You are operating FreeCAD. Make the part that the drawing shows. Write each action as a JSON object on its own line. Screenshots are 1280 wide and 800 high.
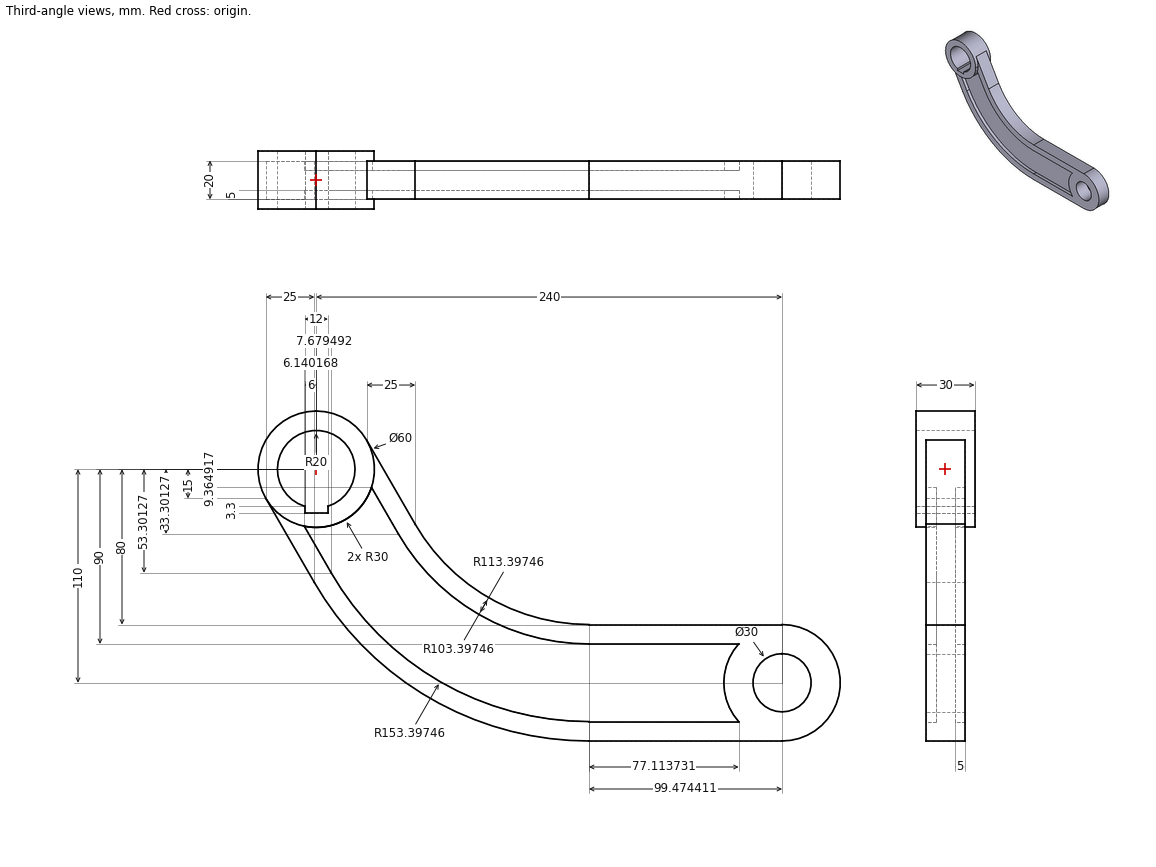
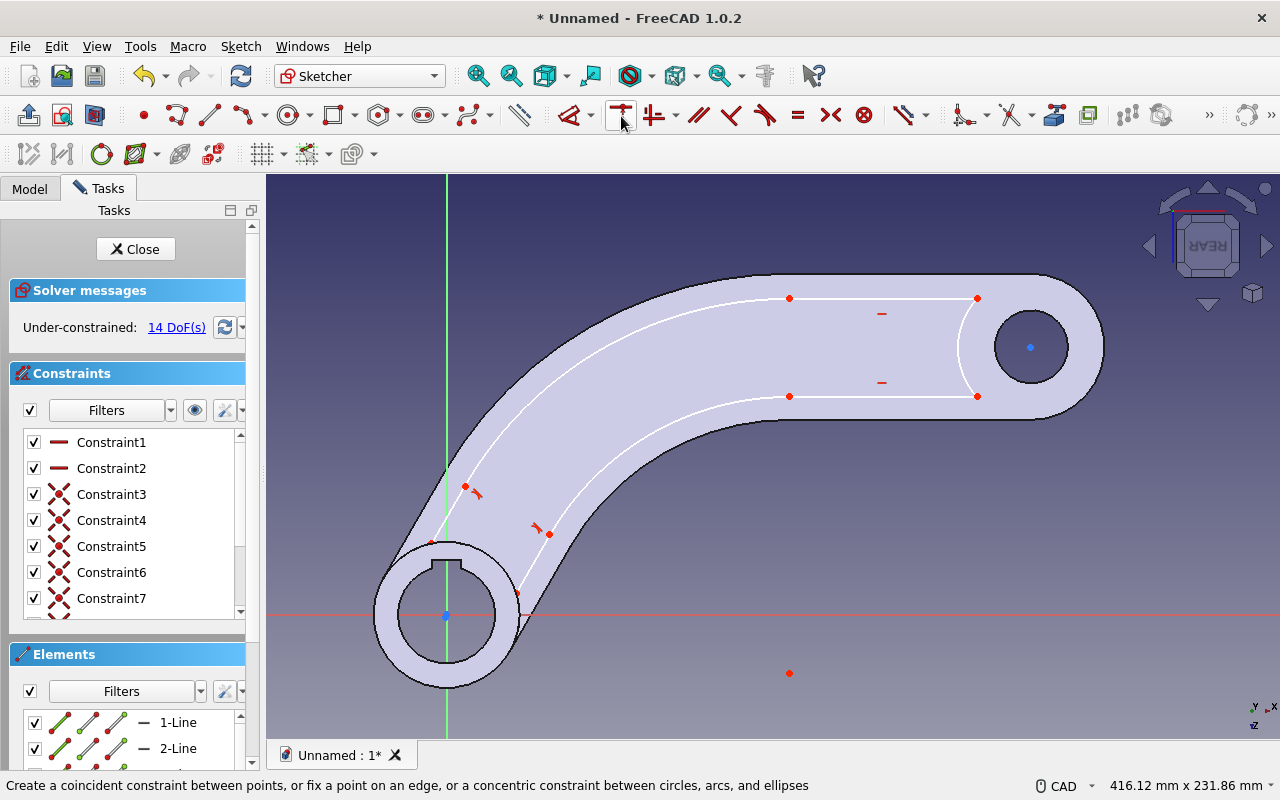
{"action": "left_click_drag", "start_coordinate": [436, 605], "coordinate": [457, 628]}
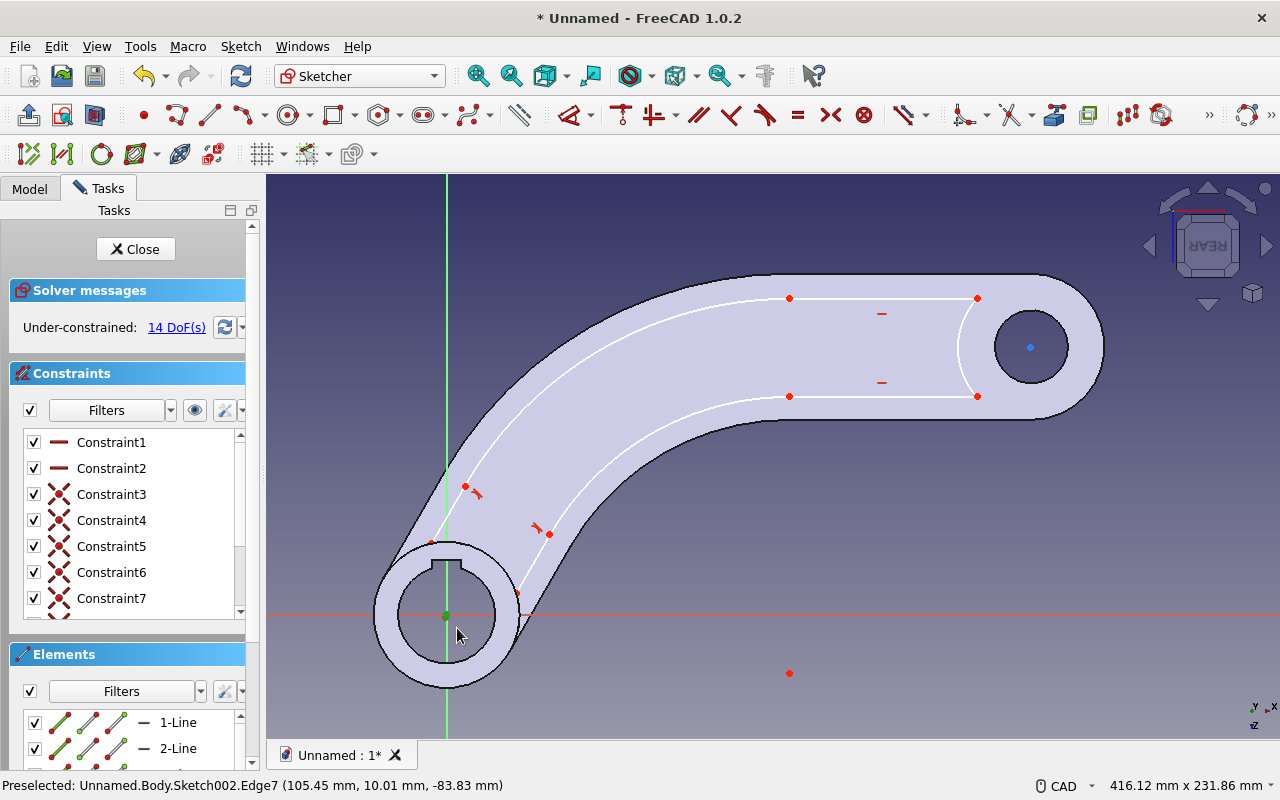
{"action": "left_click", "coordinate": [621, 116]}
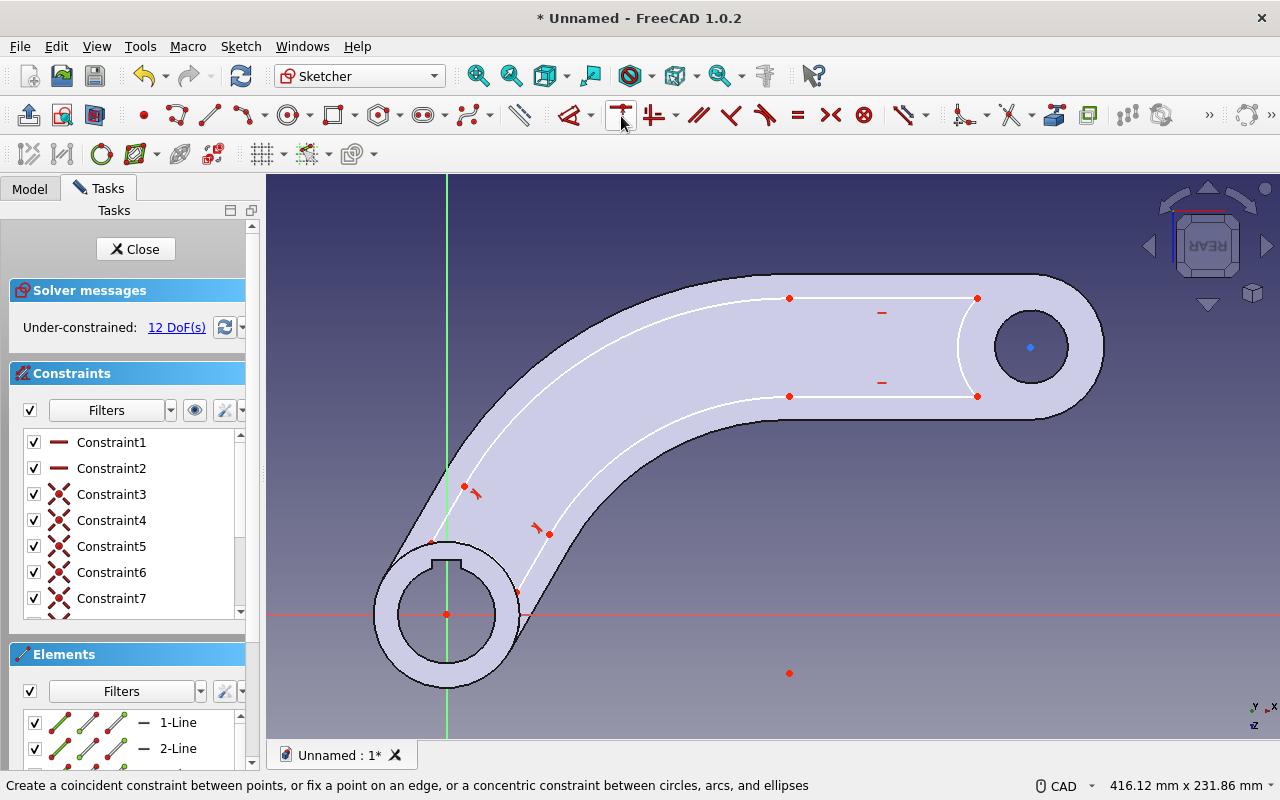
{"action": "left_click", "coordinate": [500, 565]}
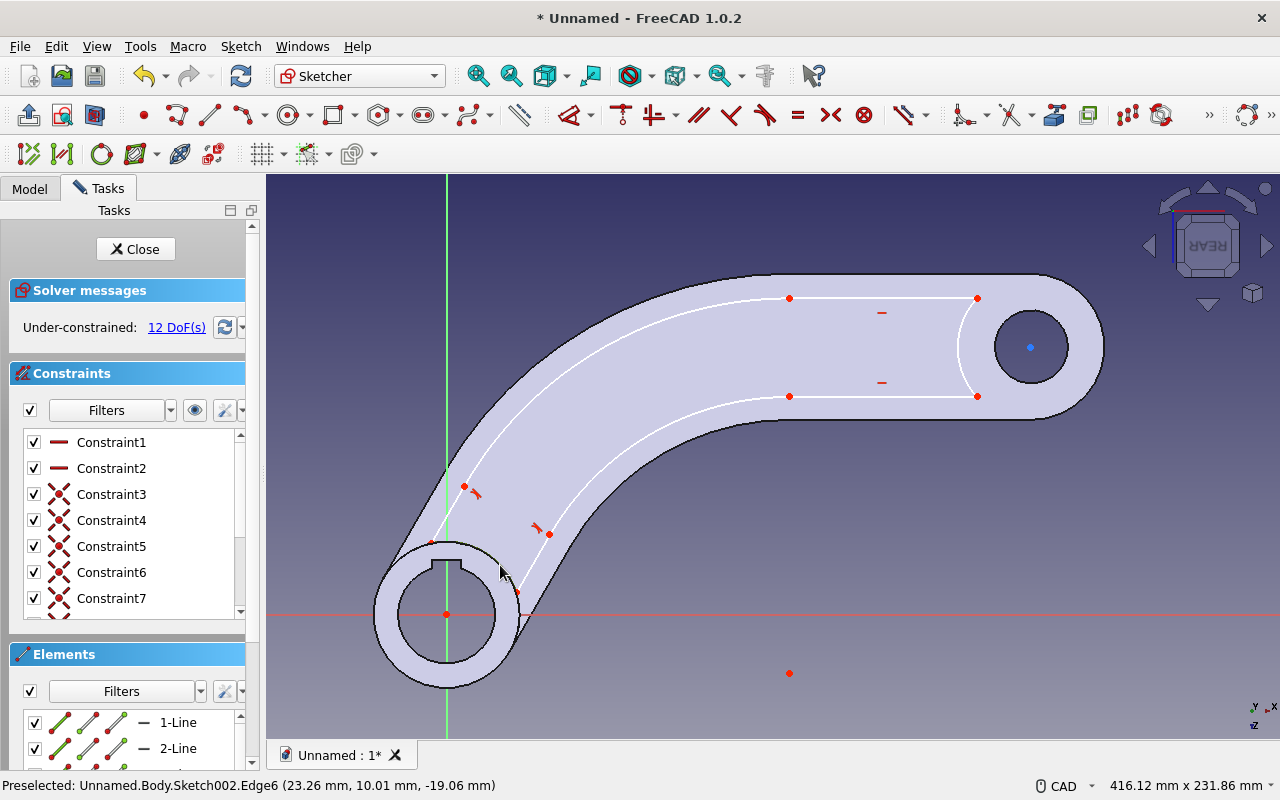
{"action": "left_click", "coordinate": [961, 326]}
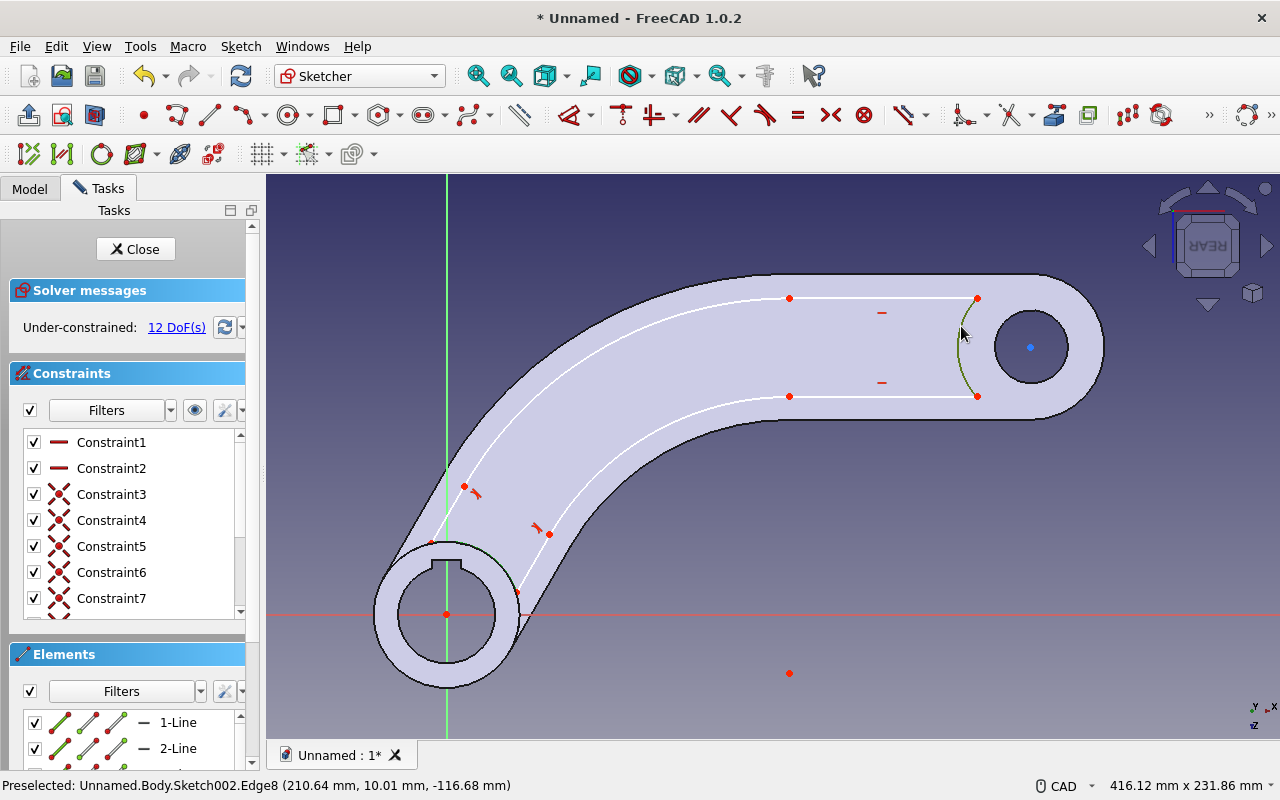
{"action": "left_click", "coordinate": [798, 116]}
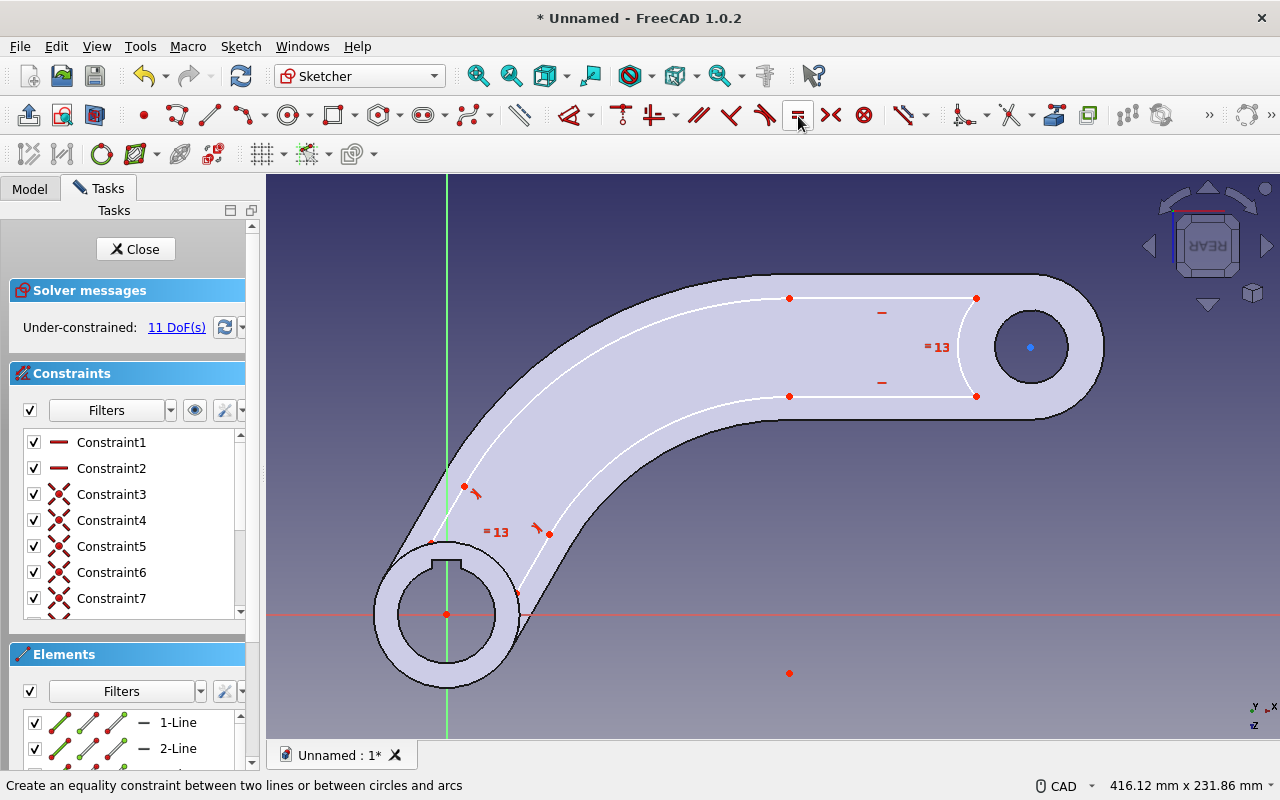
{"action": "left_click", "coordinate": [568, 116]}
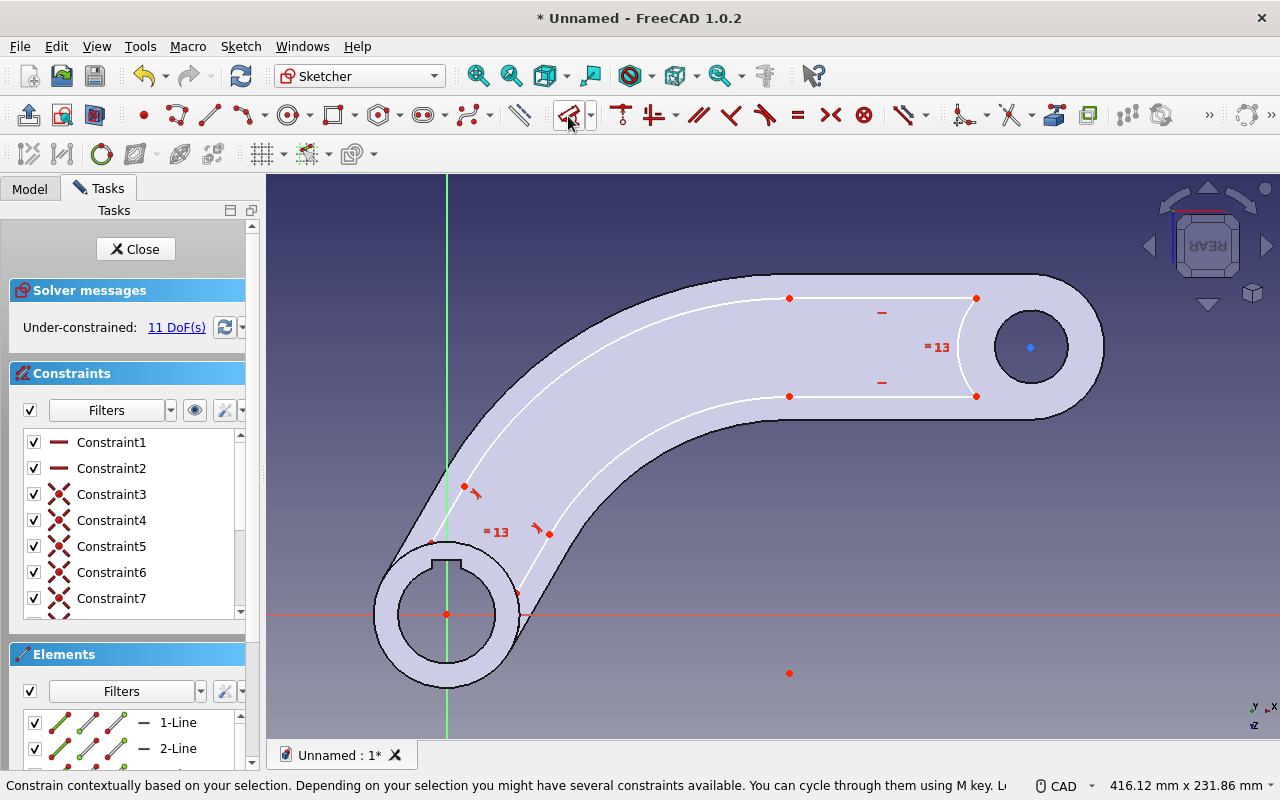
{"action": "left_click", "coordinate": [673, 317]}
{"action": "left_click", "coordinate": [663, 287]}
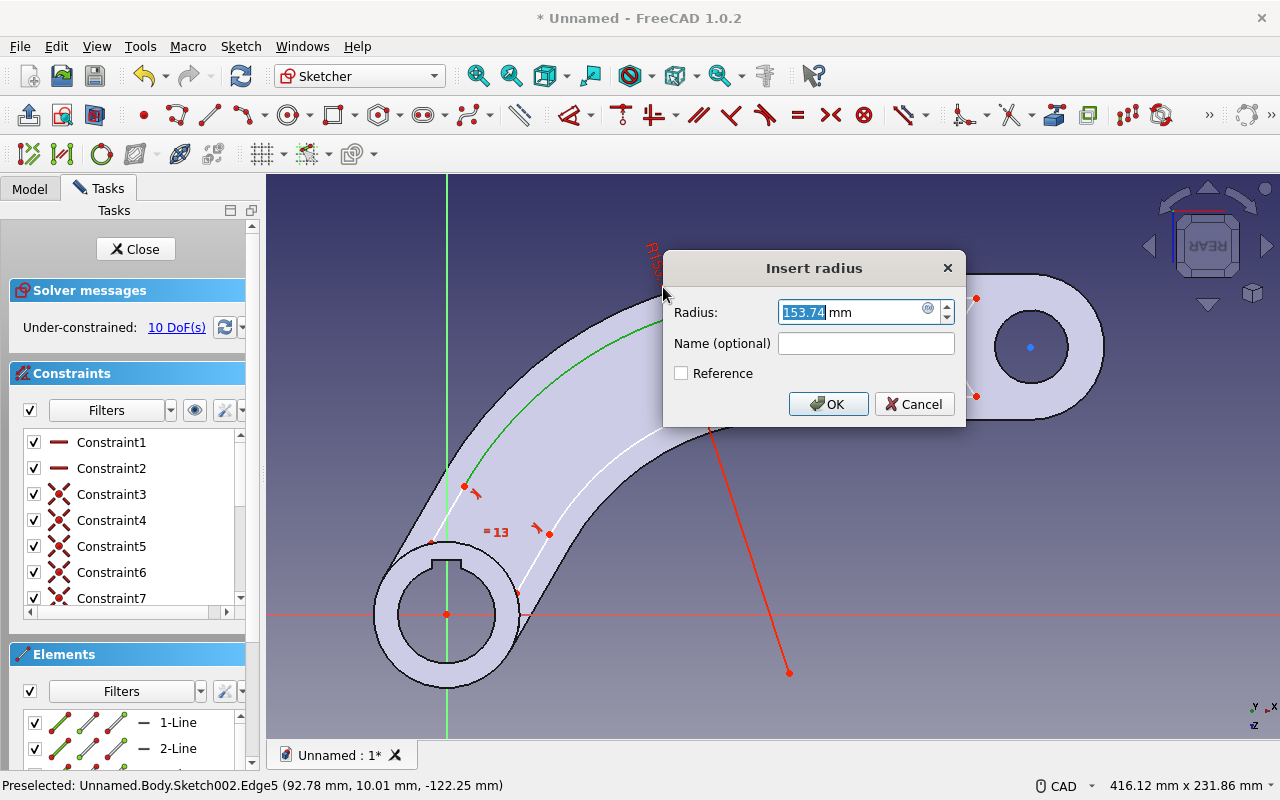
{"action": "type", "text": "153.39746"}
{"action": "key", "text": "Return"}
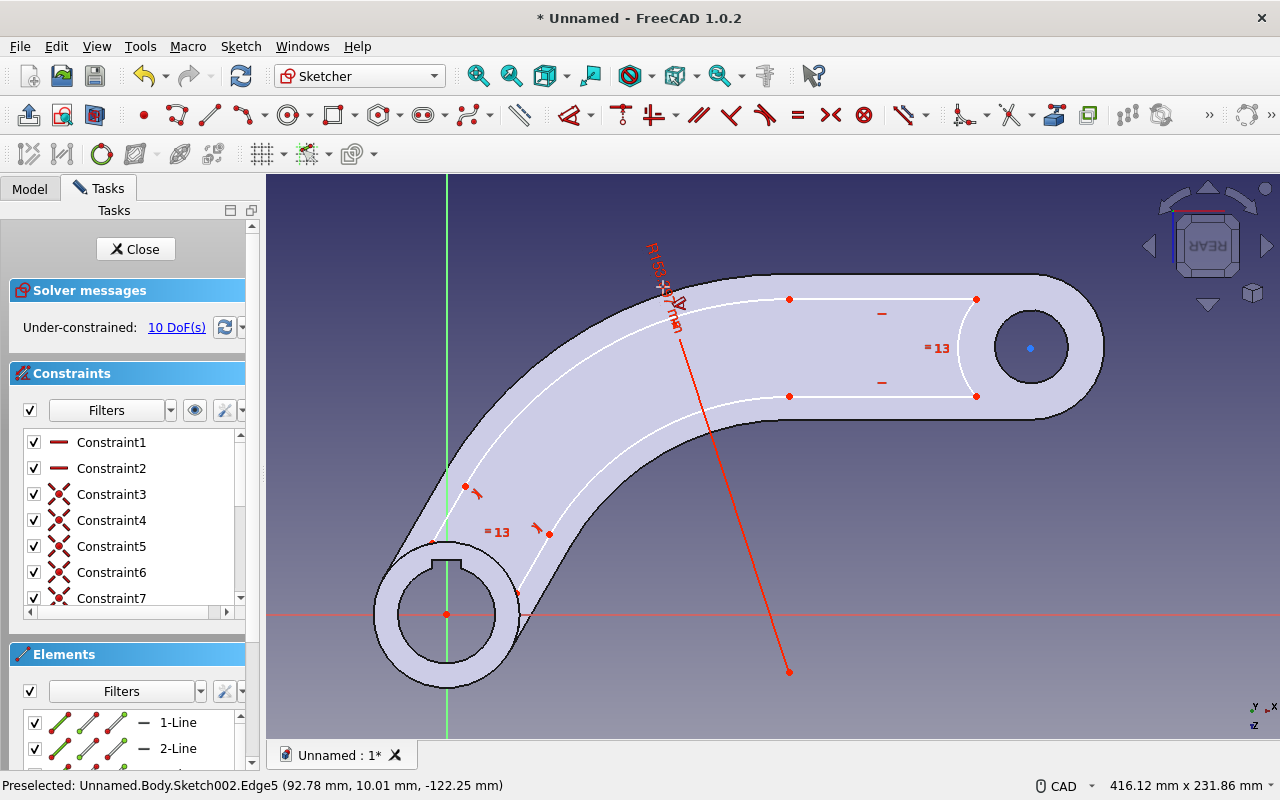
{"action": "left_click", "coordinate": [500, 566]}
{"action": "left_click", "coordinate": [524, 544]}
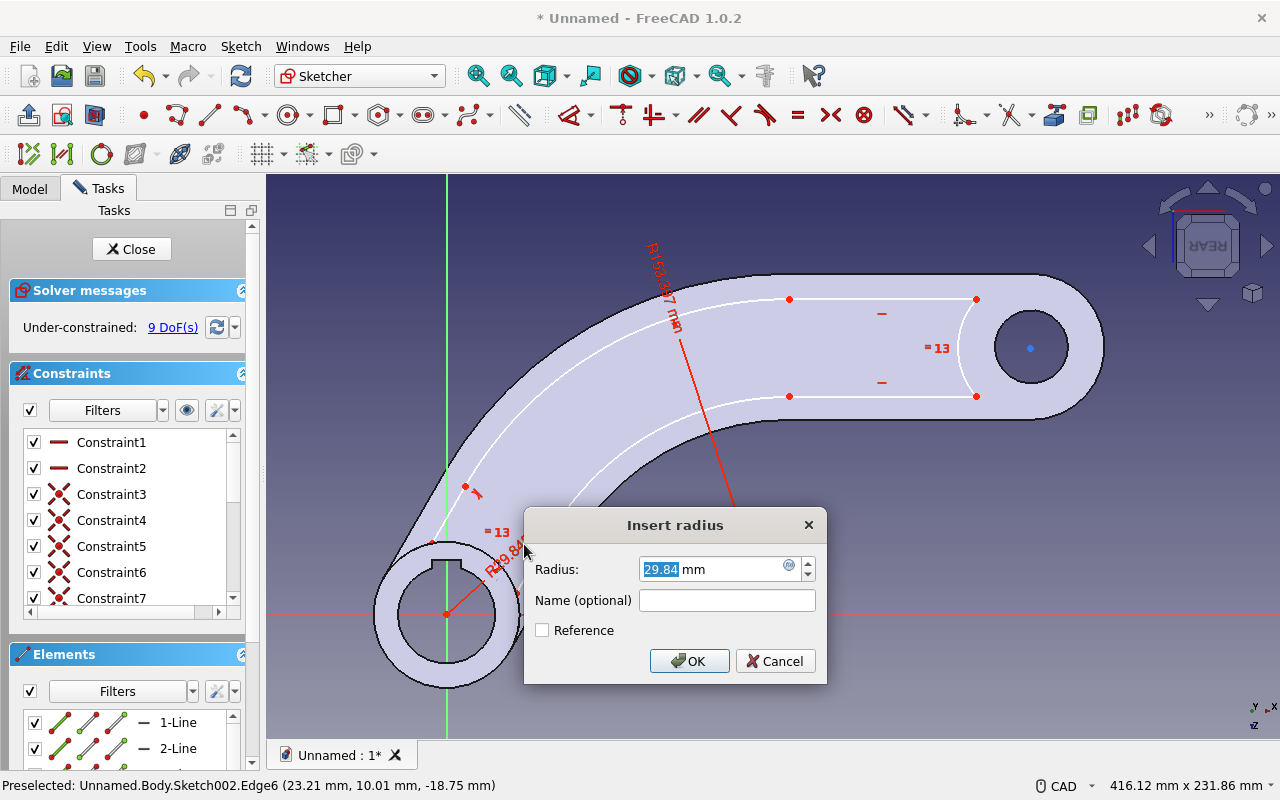
{"action": "type", "text": "30"}
{"action": "key", "text": "Return"}